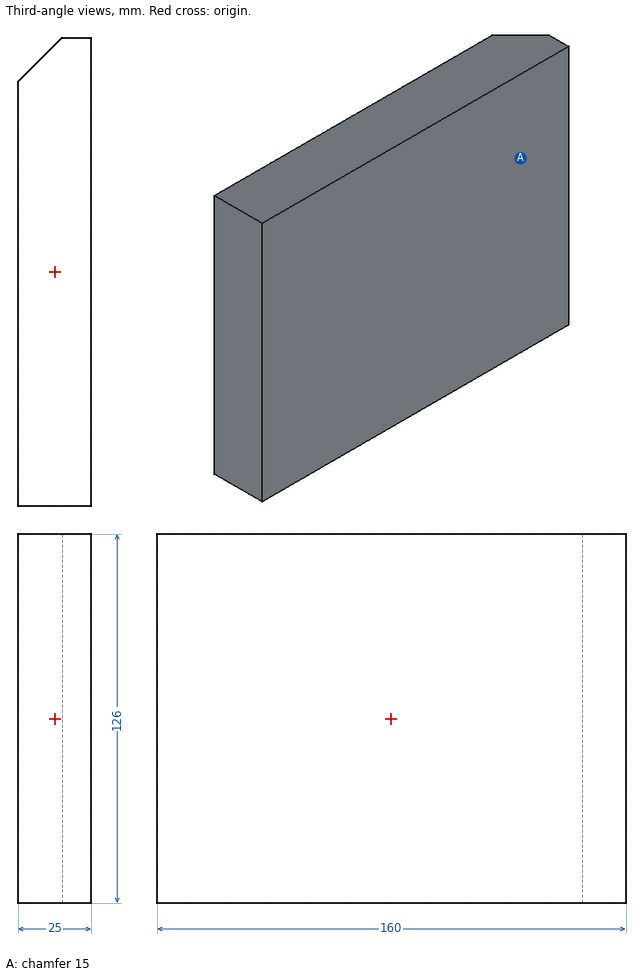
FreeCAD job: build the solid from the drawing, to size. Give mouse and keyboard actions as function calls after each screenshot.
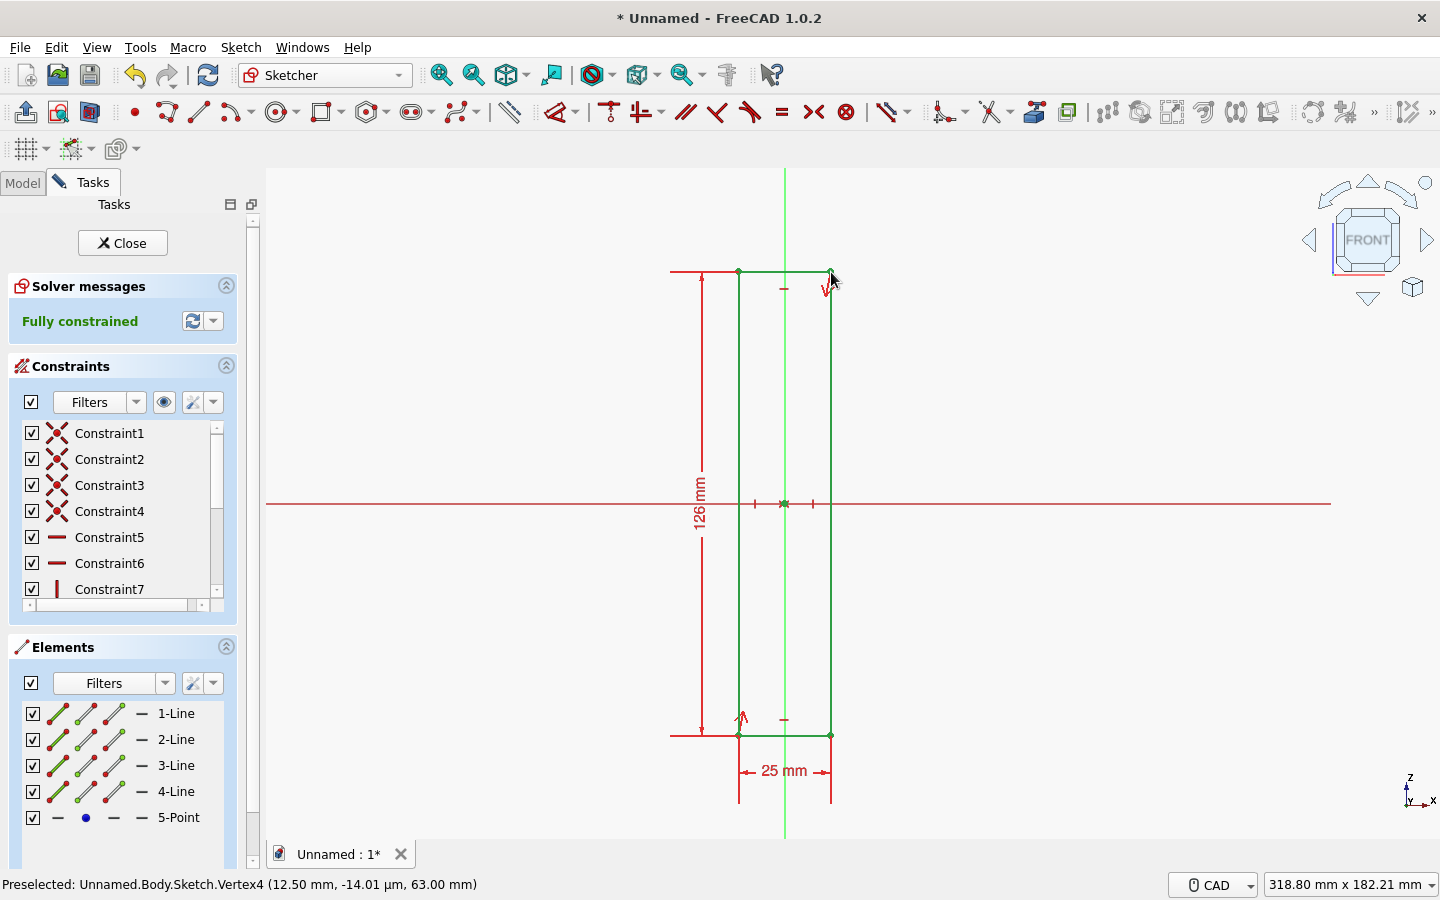
click(123, 243)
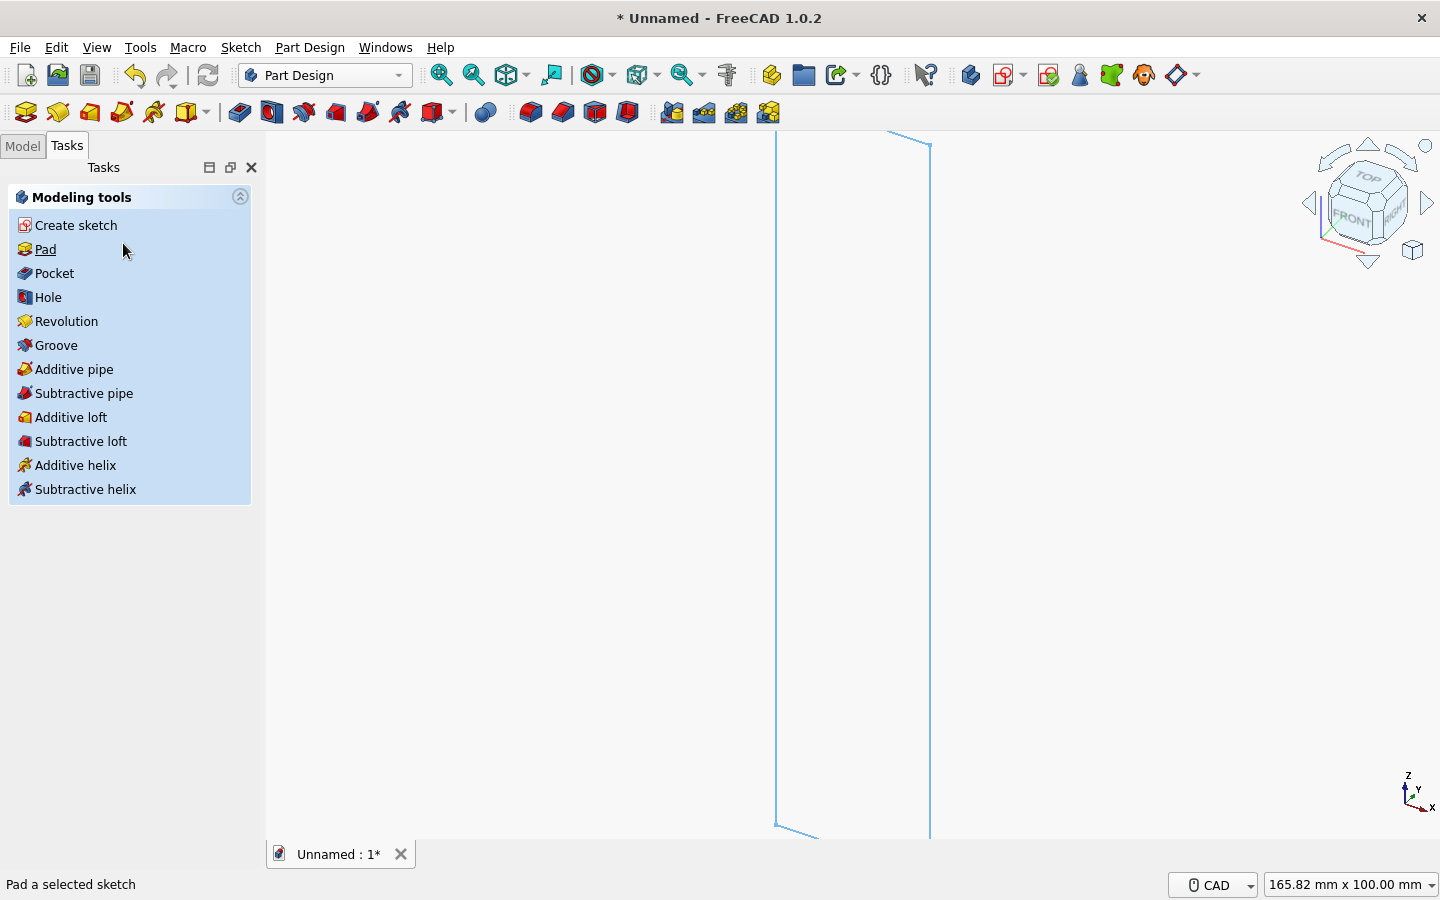
click(26, 112)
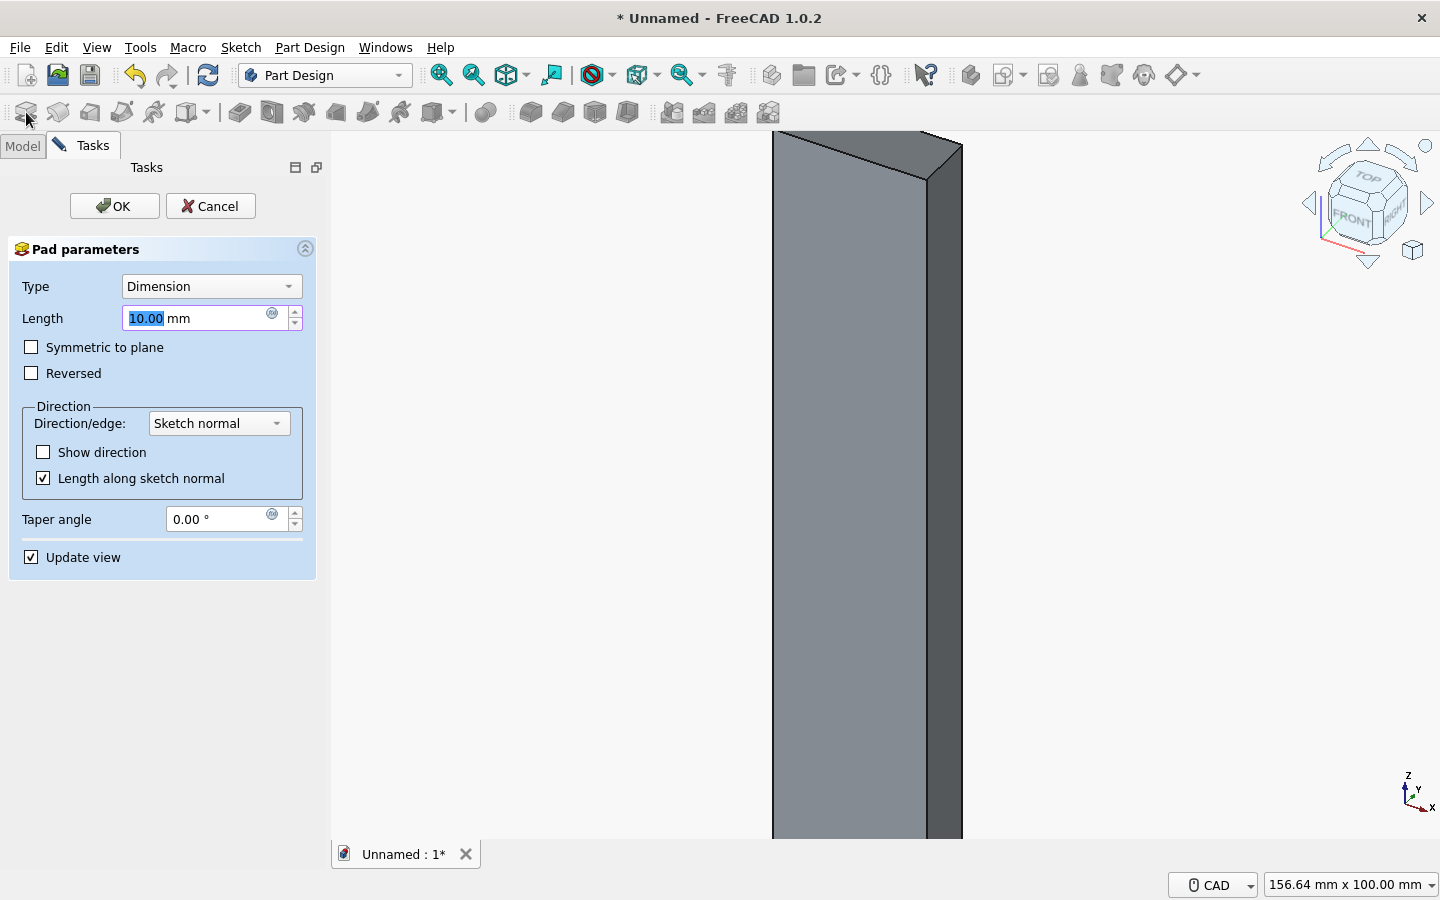
text(160)
key(Tab)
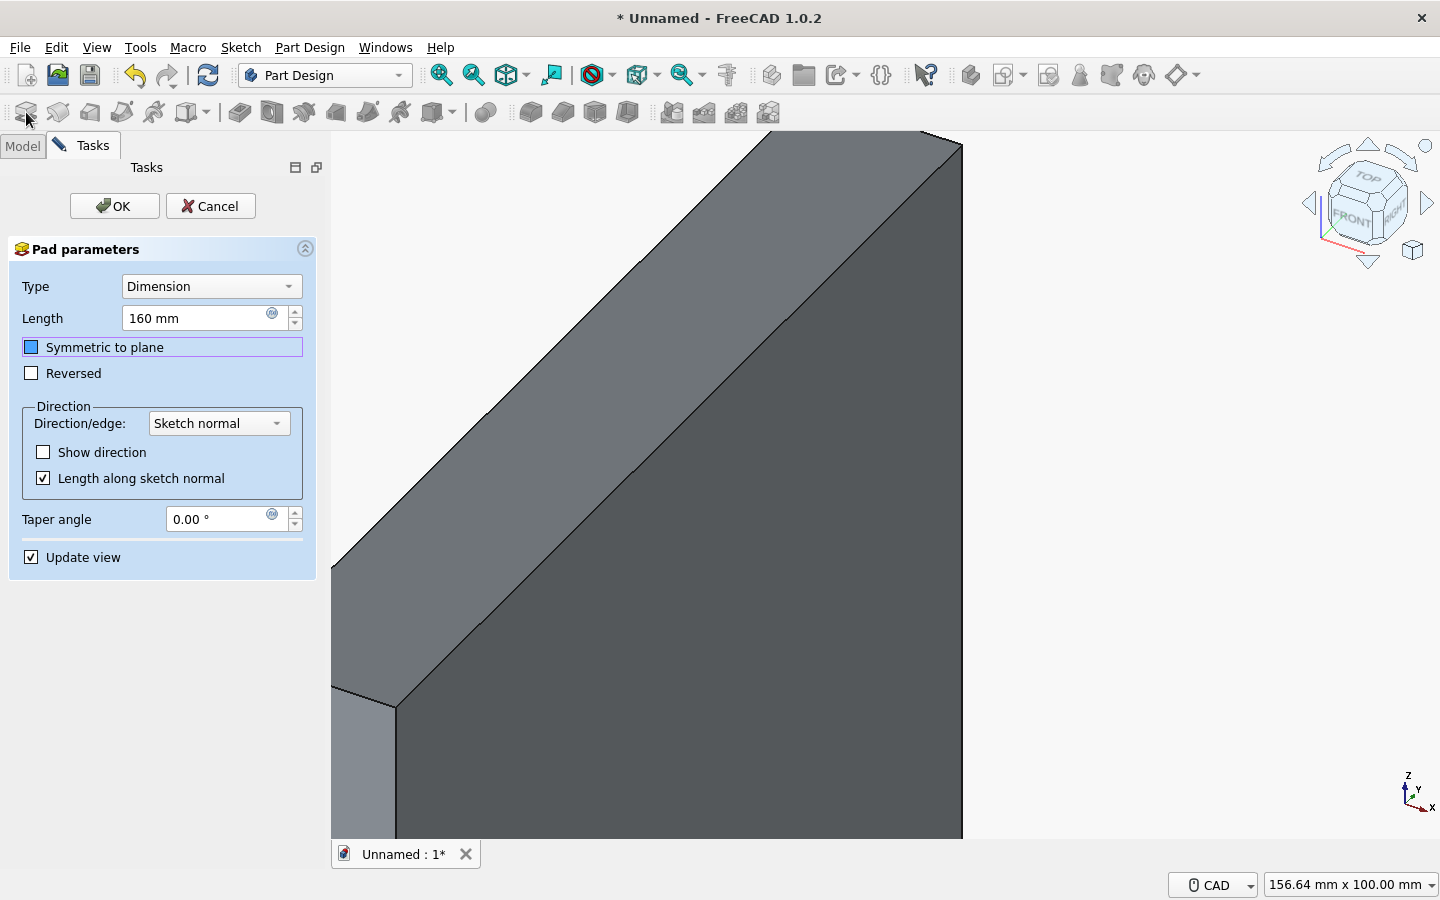
click(30, 347)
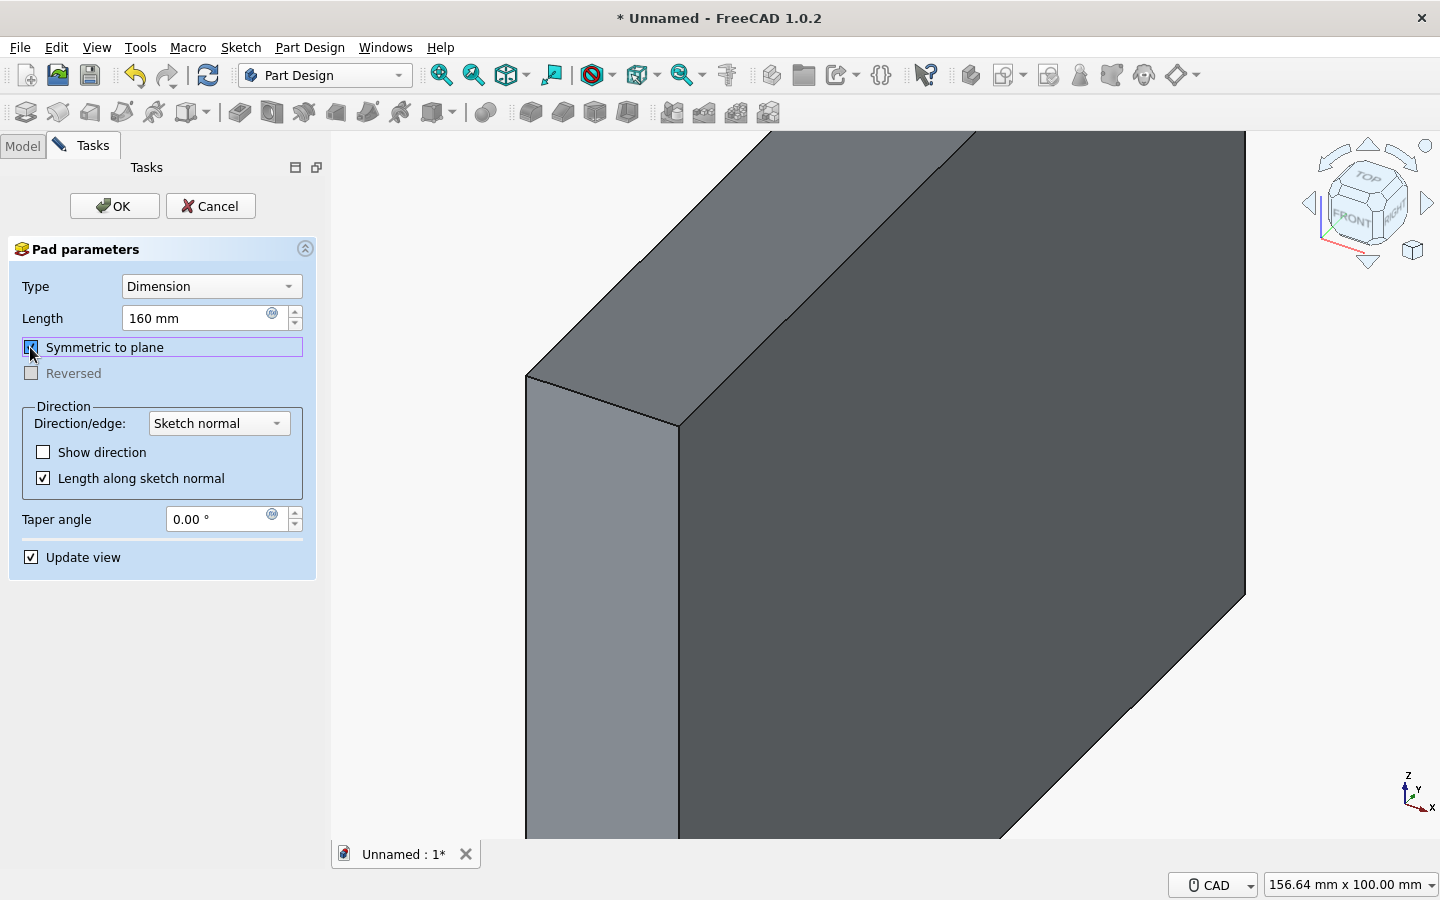
click(115, 206)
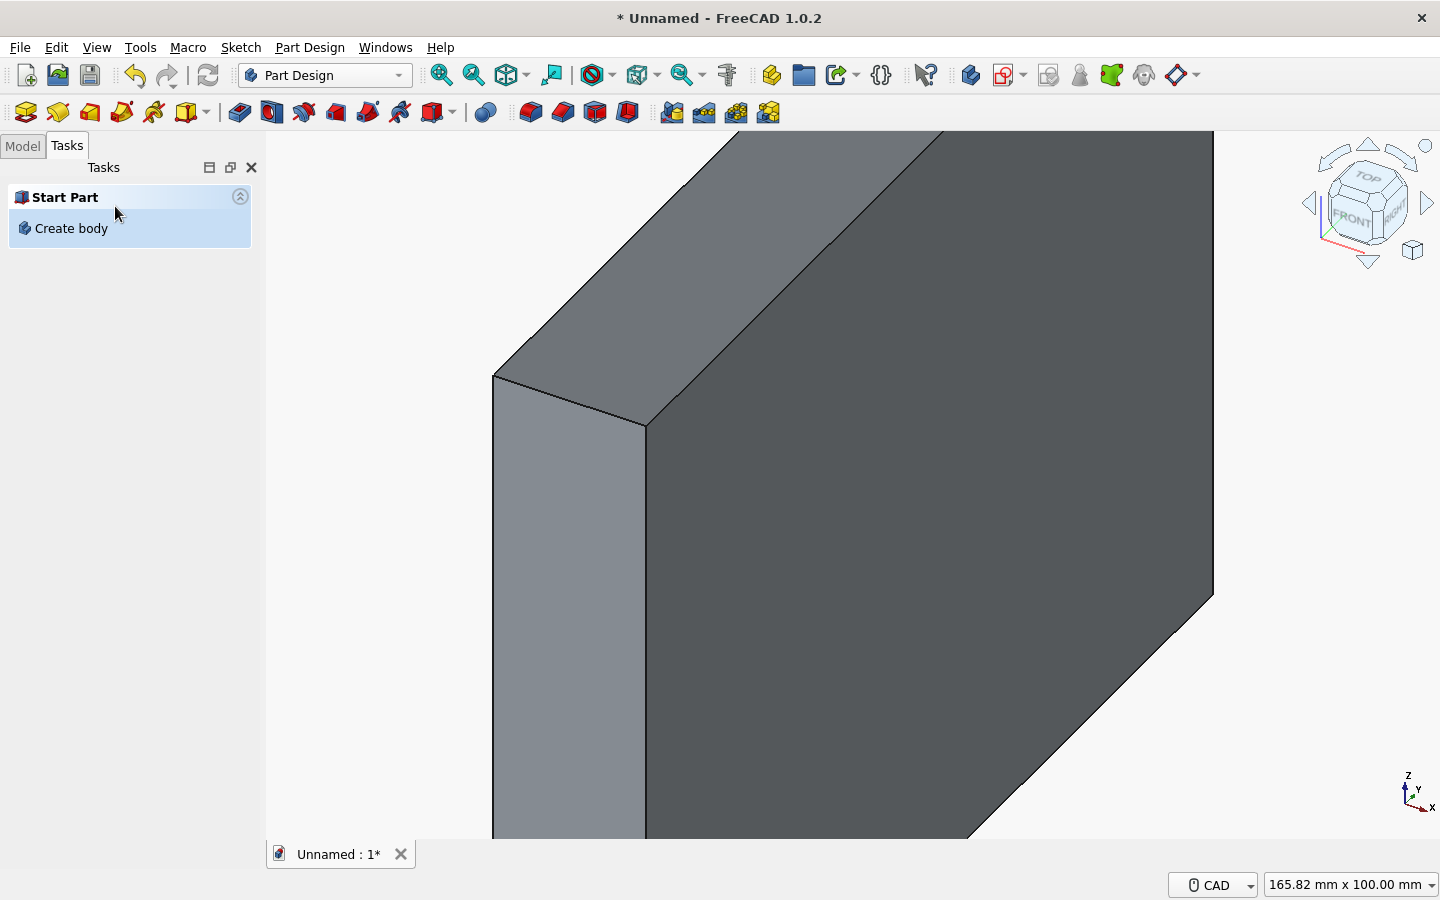
click(442, 76)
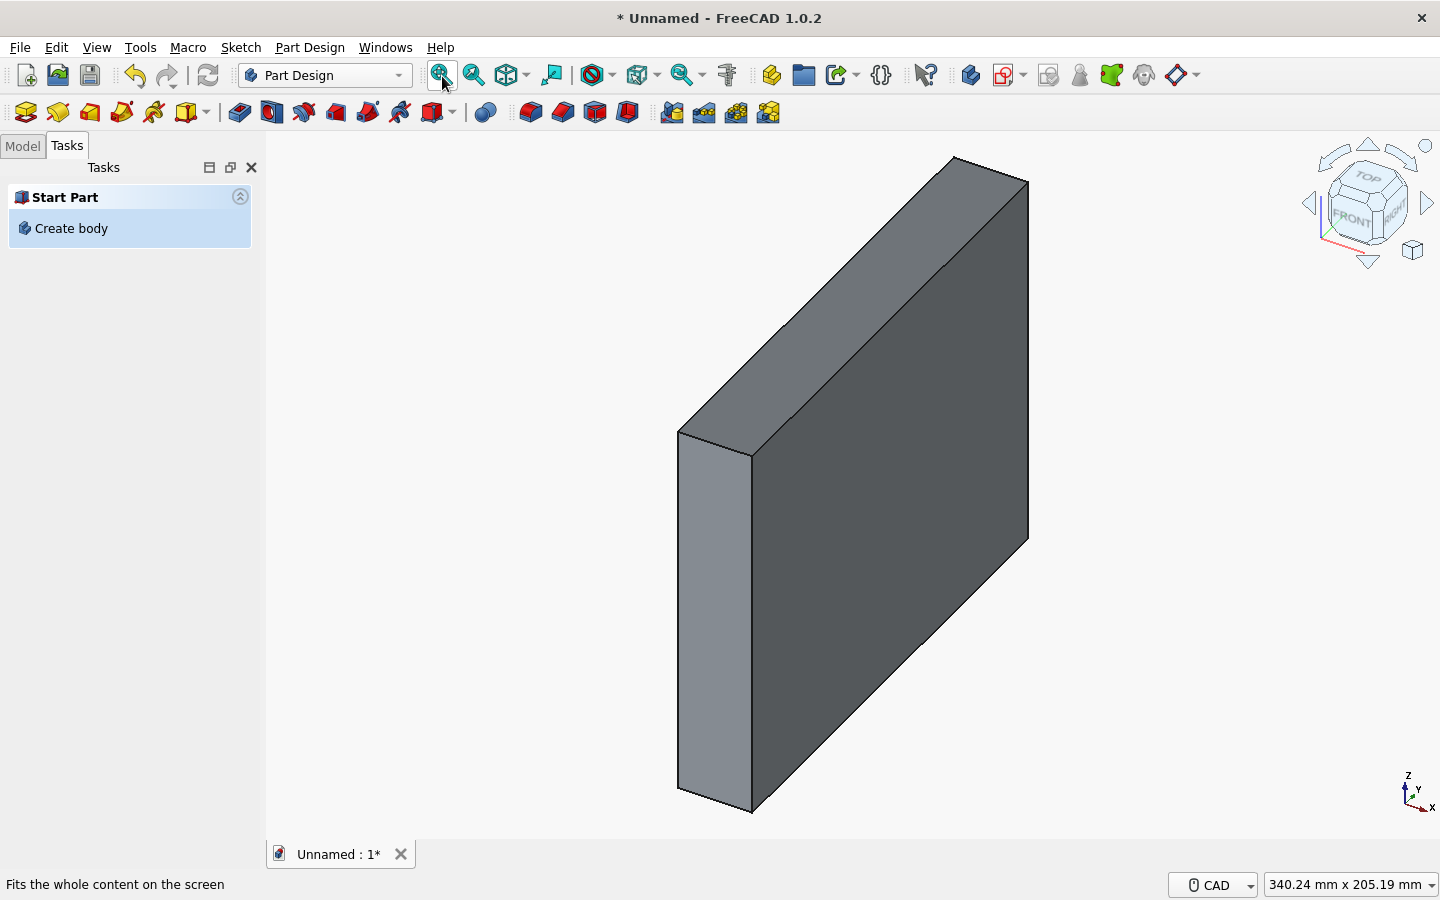
key(0)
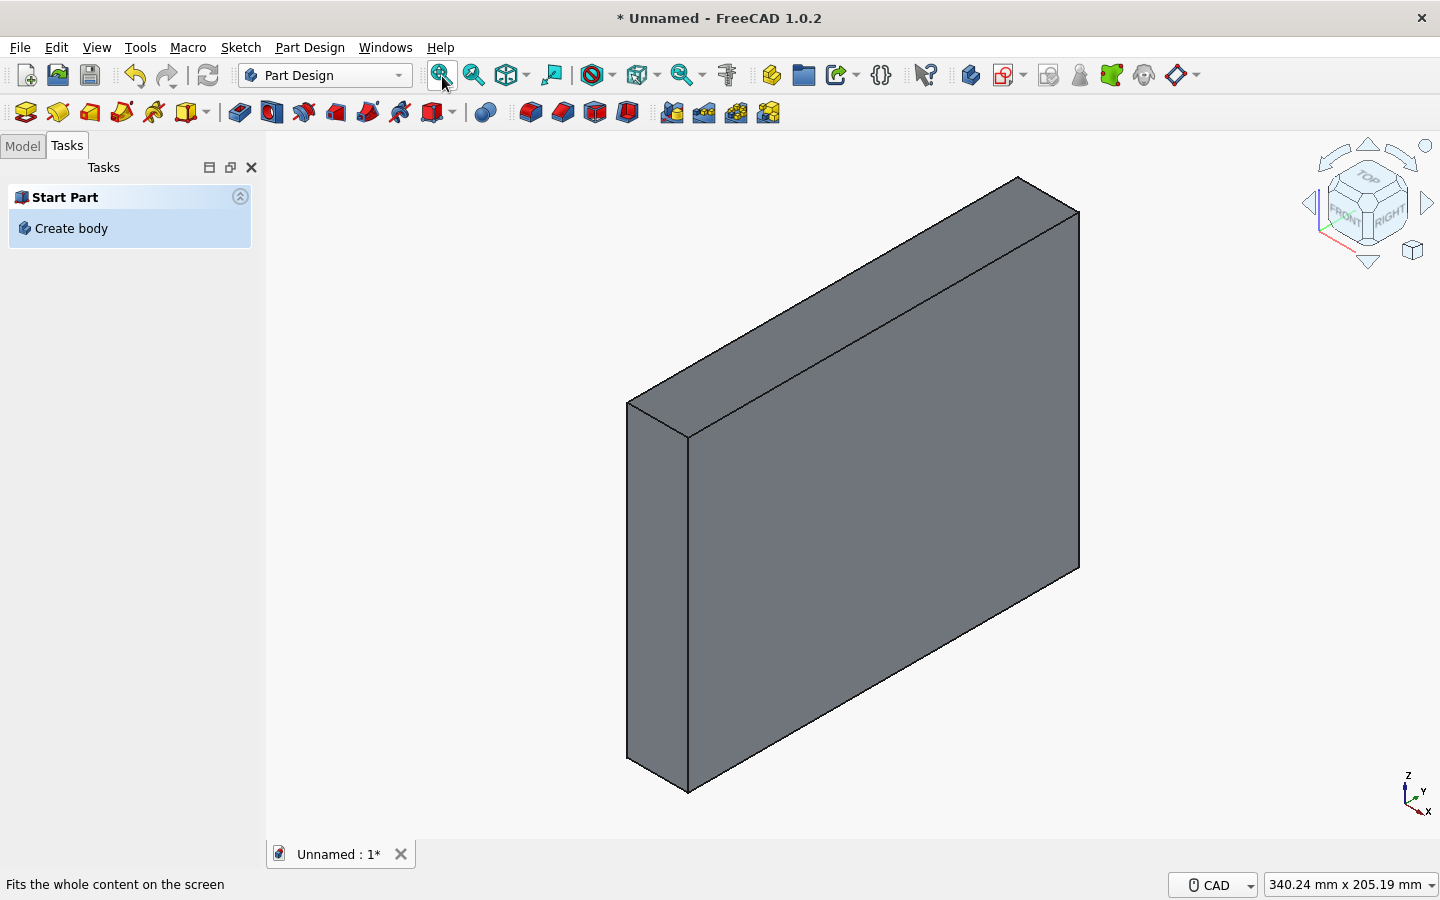
key(2)